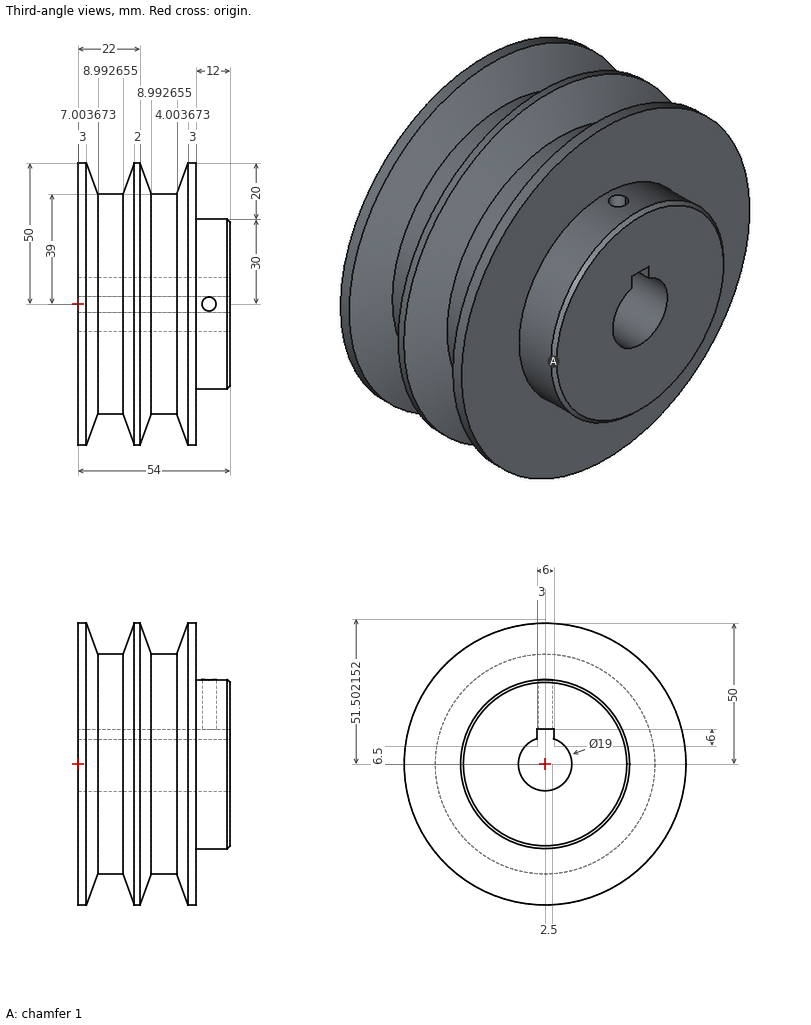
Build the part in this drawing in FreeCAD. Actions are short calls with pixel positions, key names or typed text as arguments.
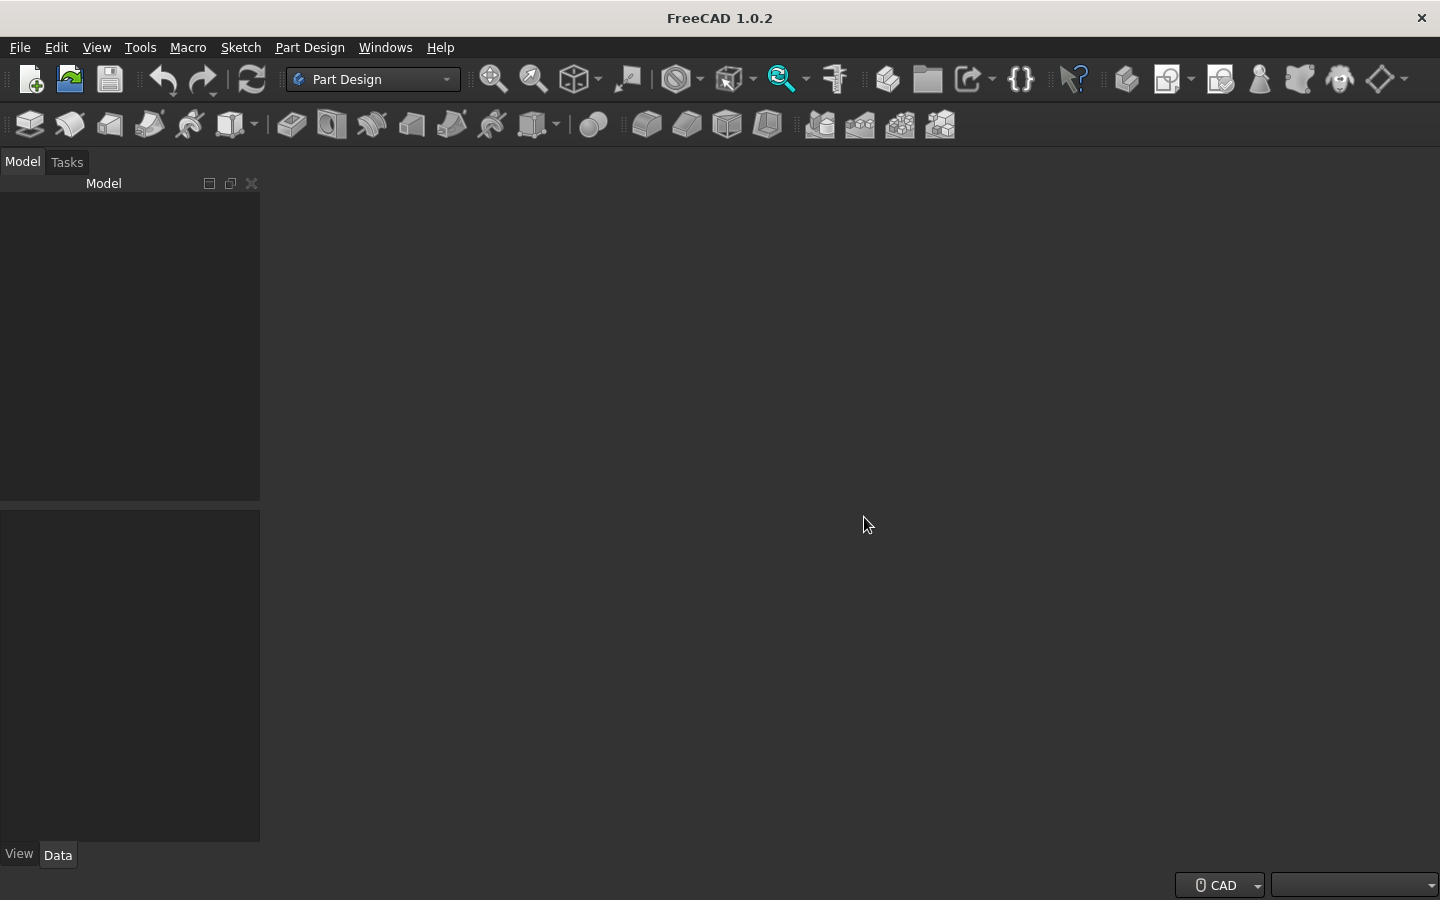
click(30, 80)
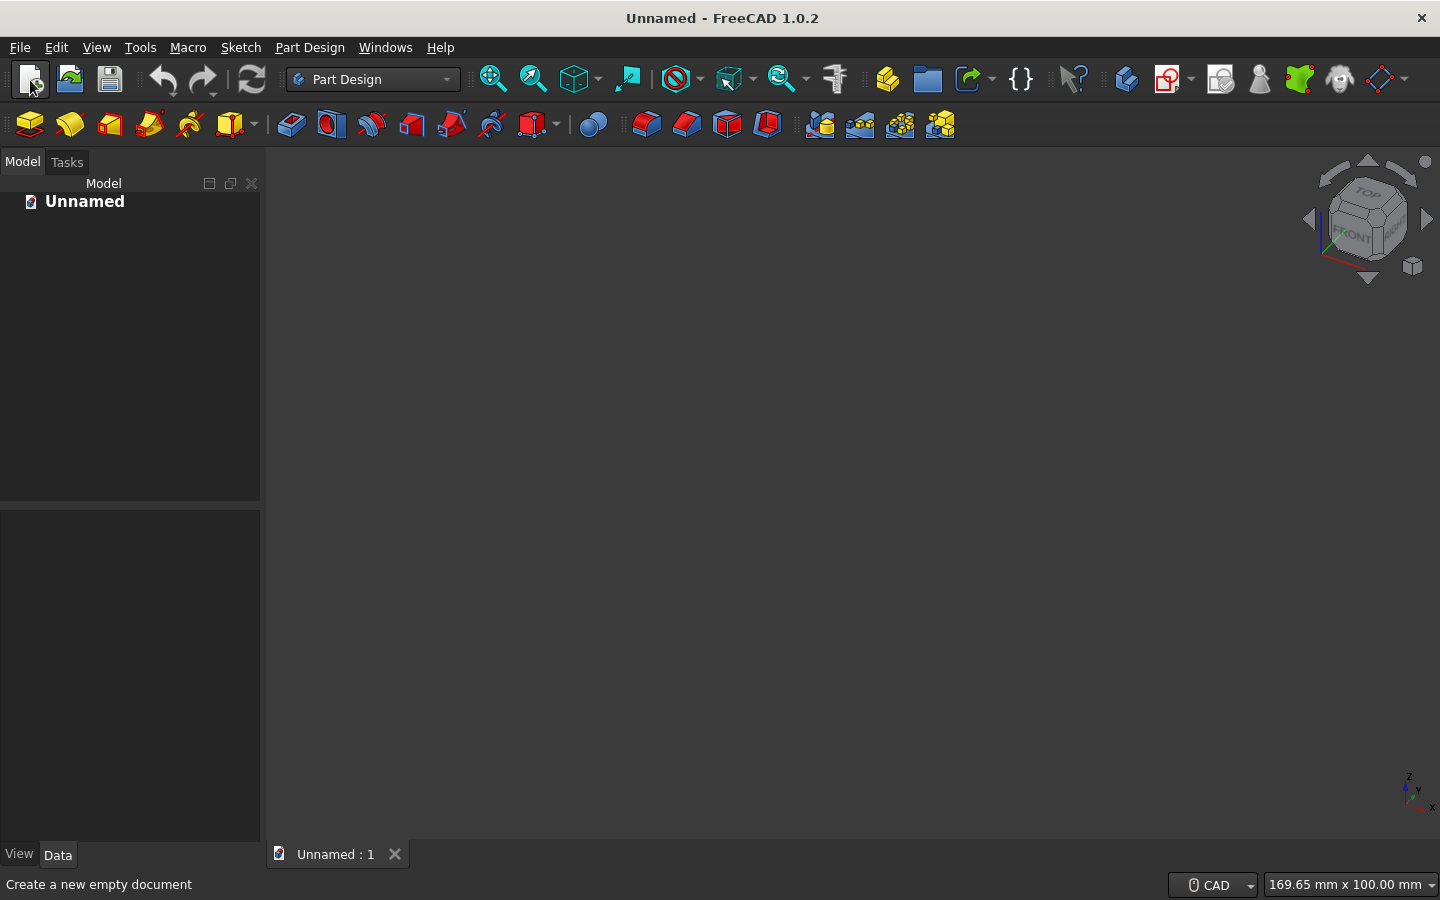
click(1168, 80)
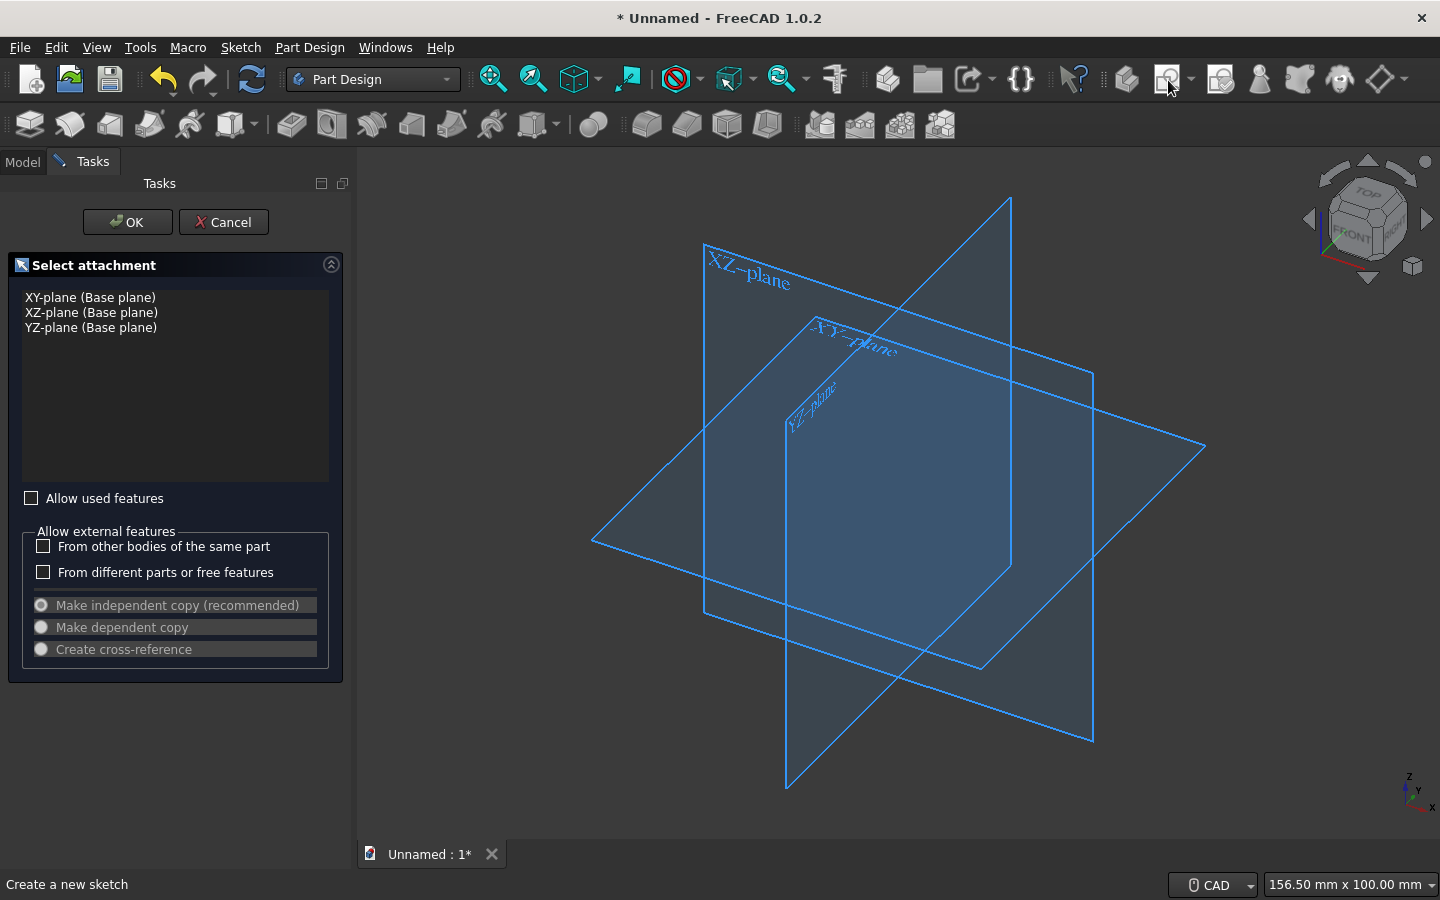
click(82, 298)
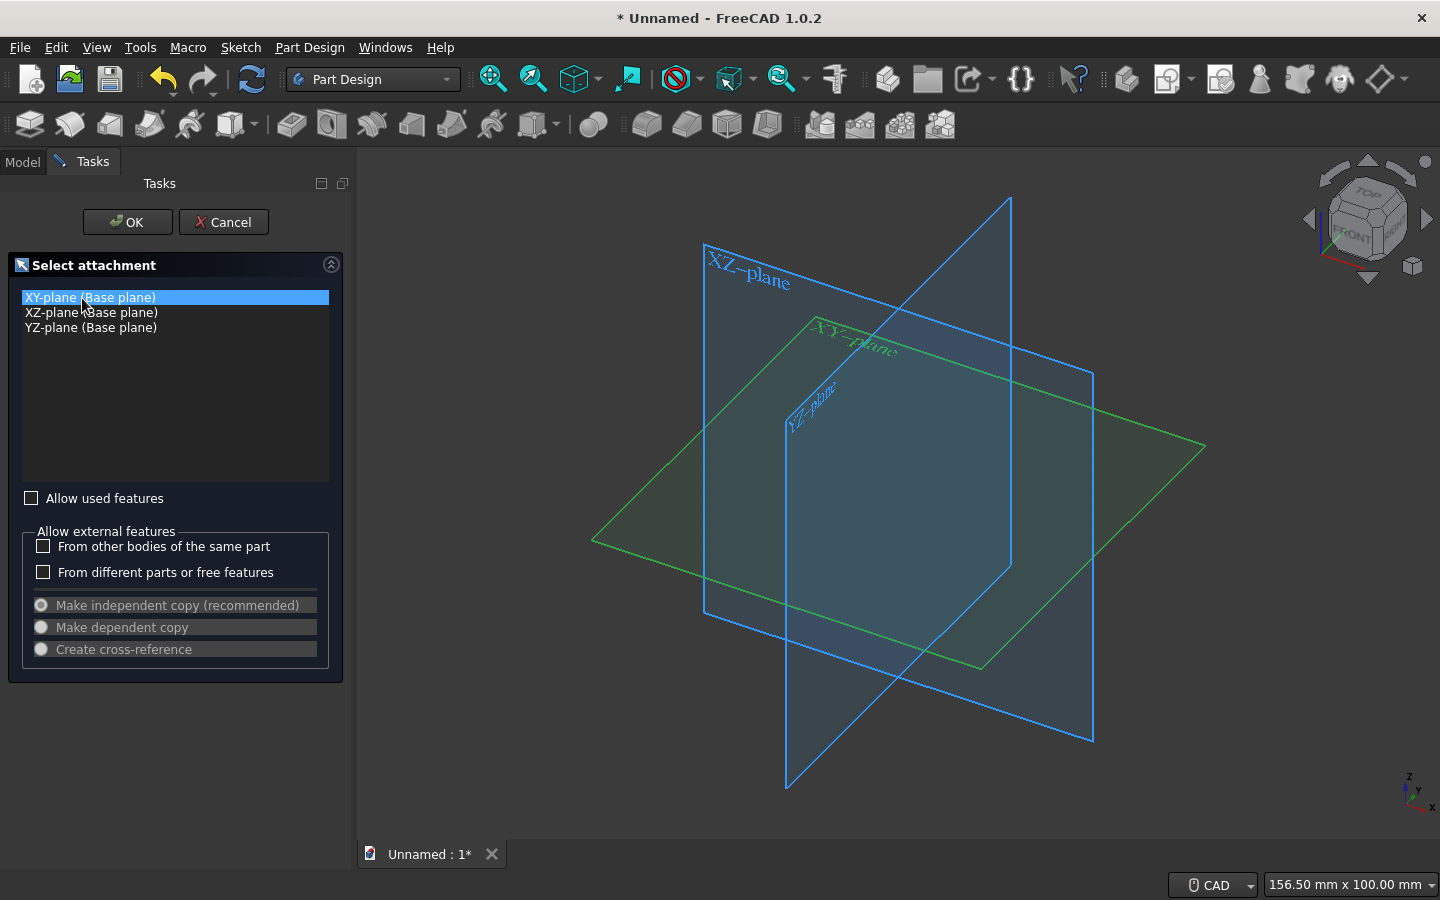
click(128, 222)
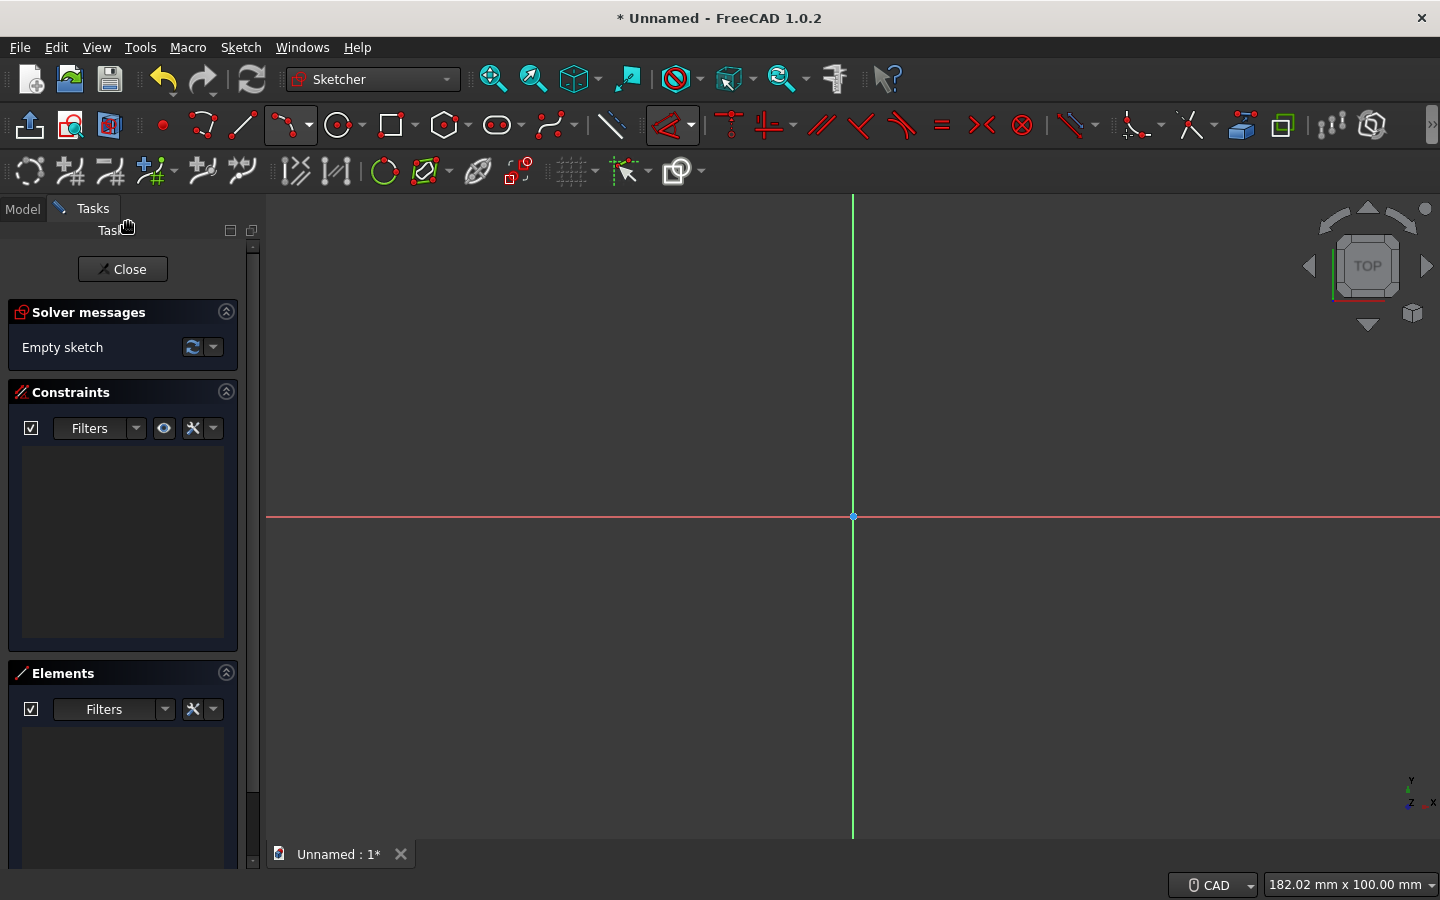
scroll(294, 811, down, 1)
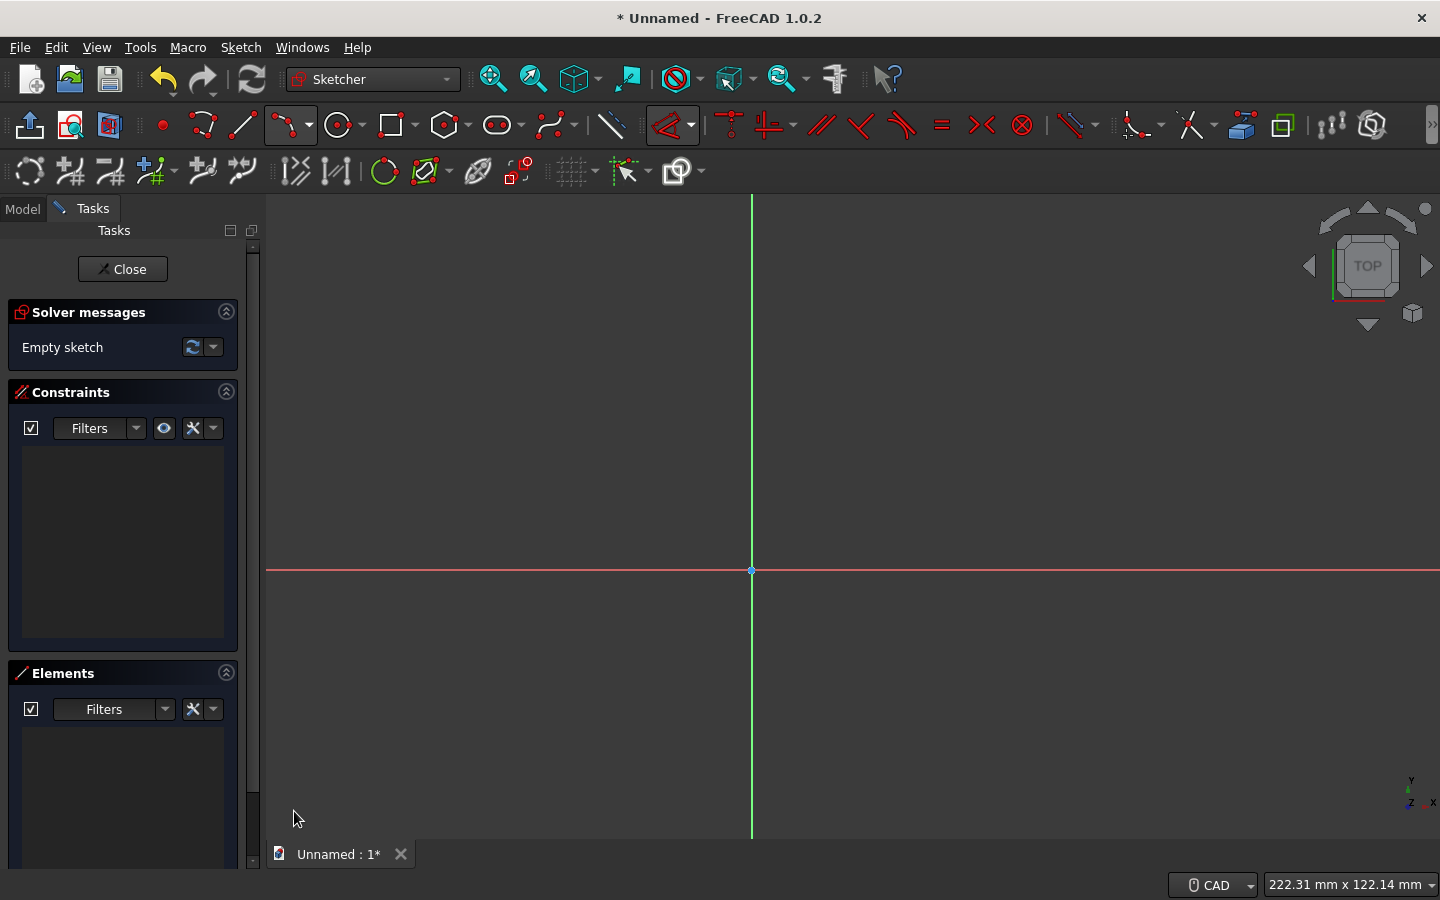
scroll(1117, 279, up, 2)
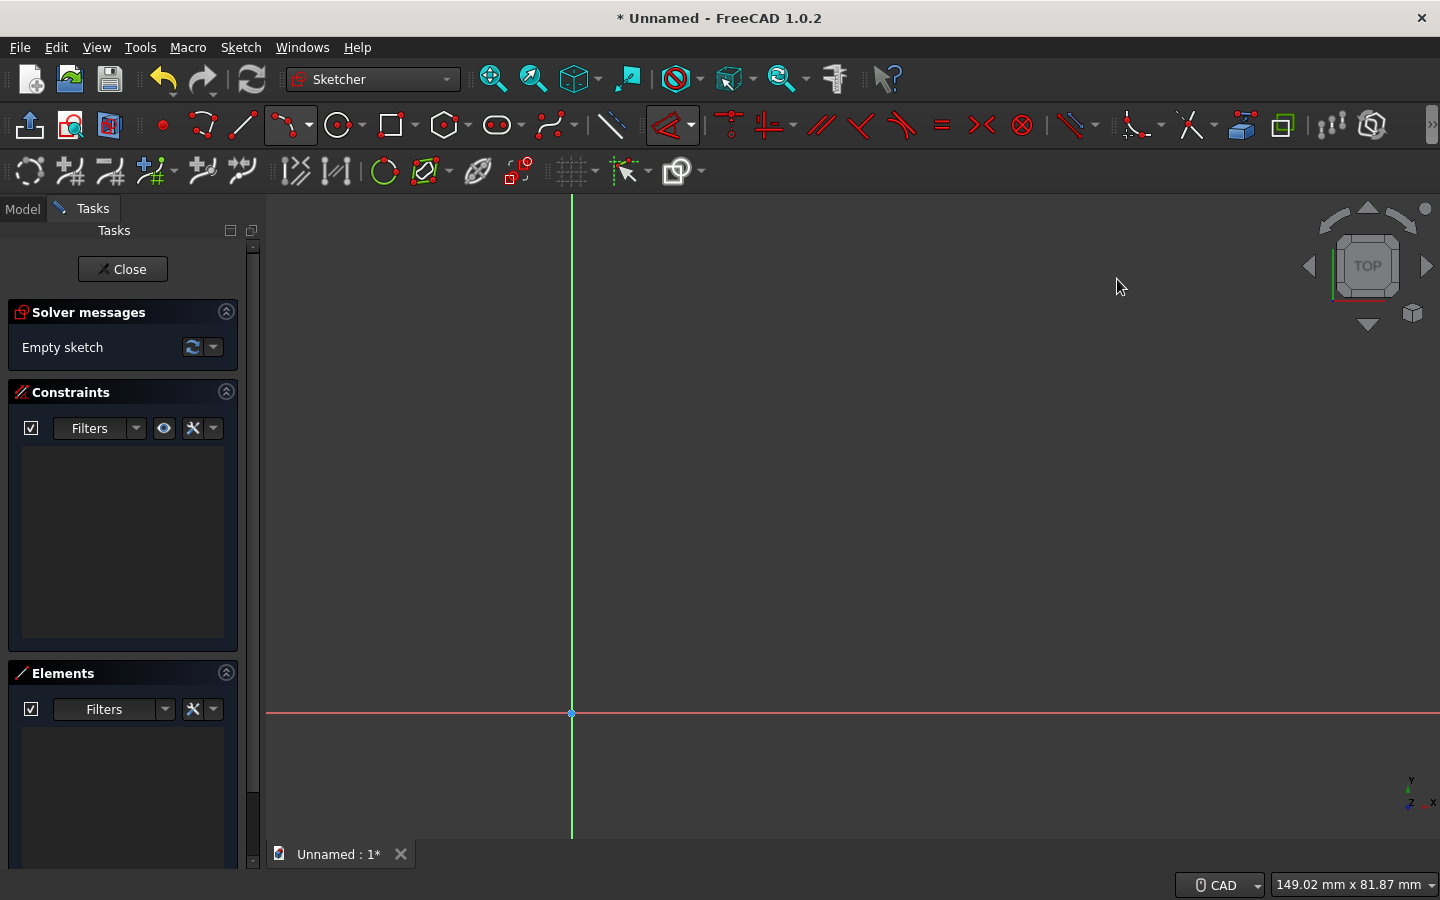
click(204, 126)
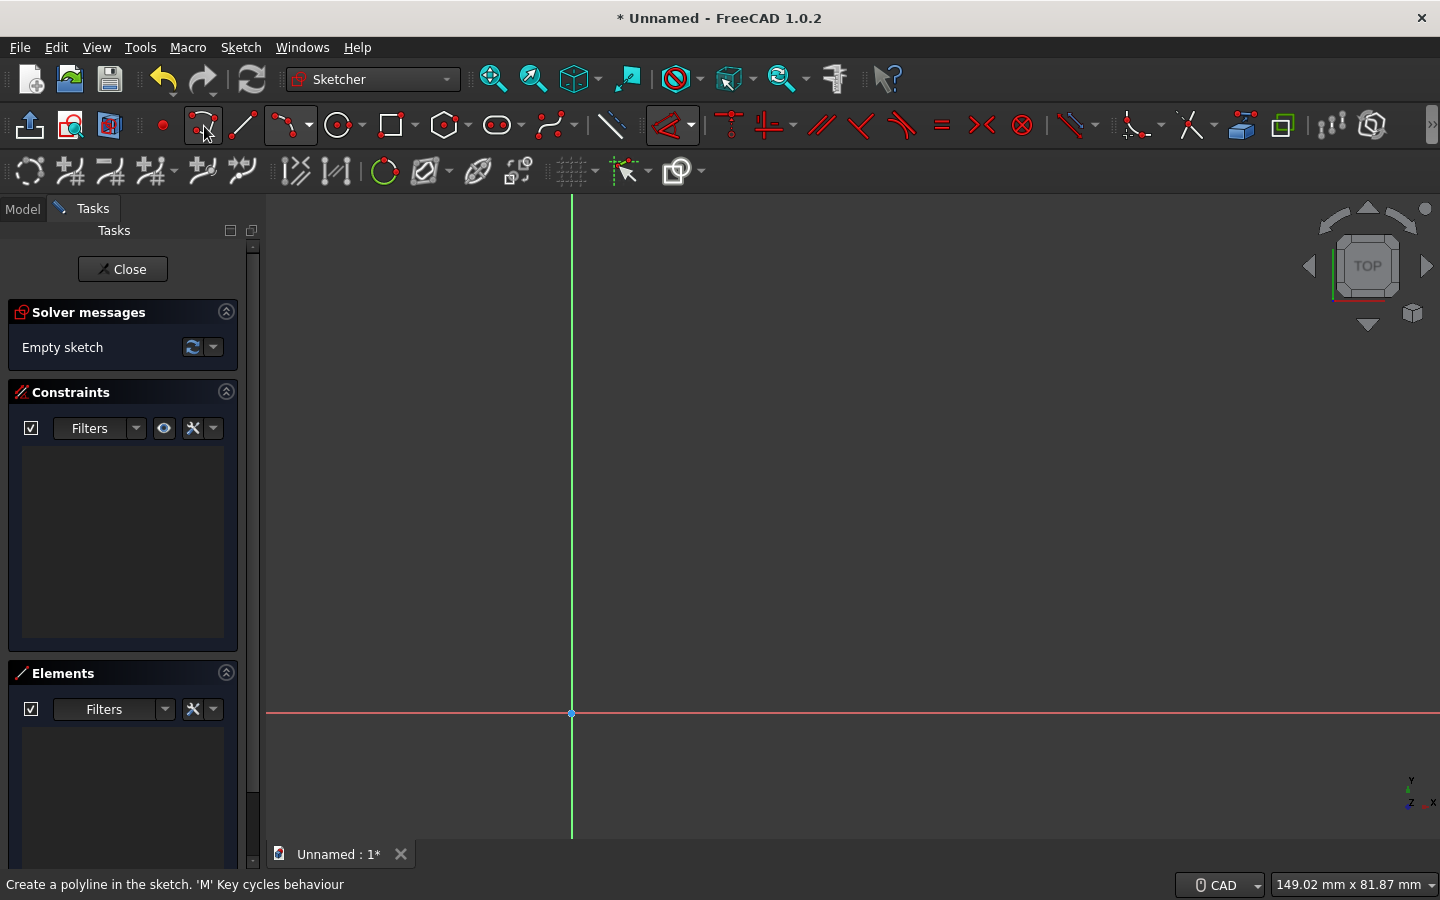
click(572, 713)
click(997, 704)
click(997, 477)
click(903, 477)
click(903, 319)
click(879, 319)
click(847, 406)
click(777, 406)
click(745, 319)
click(729, 319)
click(698, 406)
click(627, 406)
click(595, 319)
click(581, 319)
click(572, 713)
key(Escape)
key(Escape)